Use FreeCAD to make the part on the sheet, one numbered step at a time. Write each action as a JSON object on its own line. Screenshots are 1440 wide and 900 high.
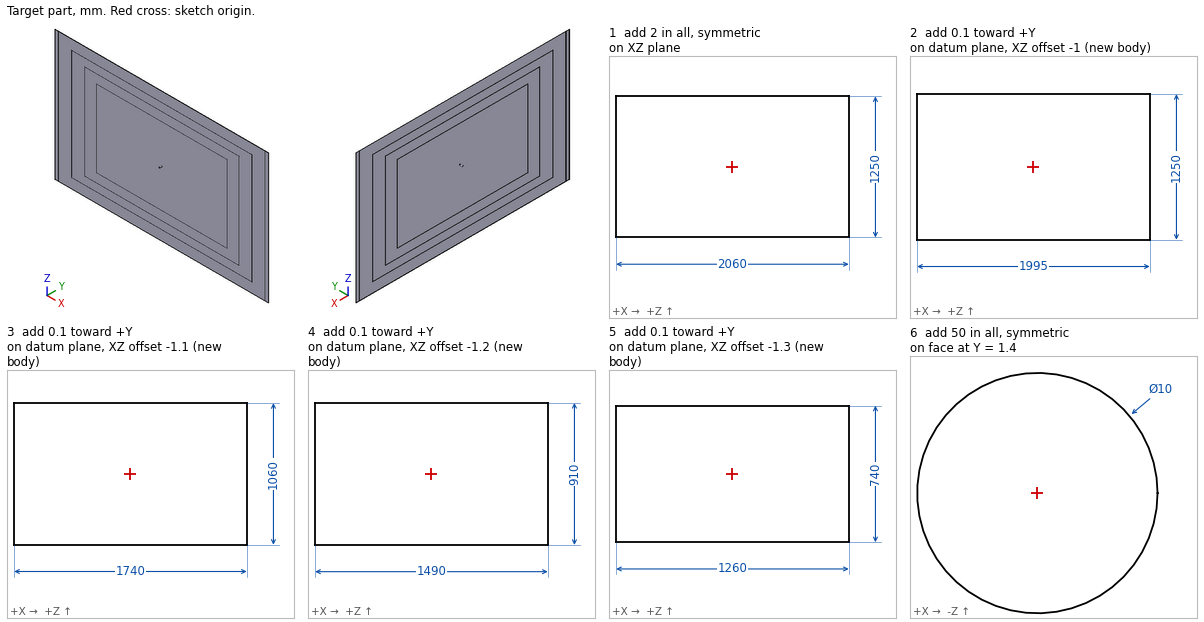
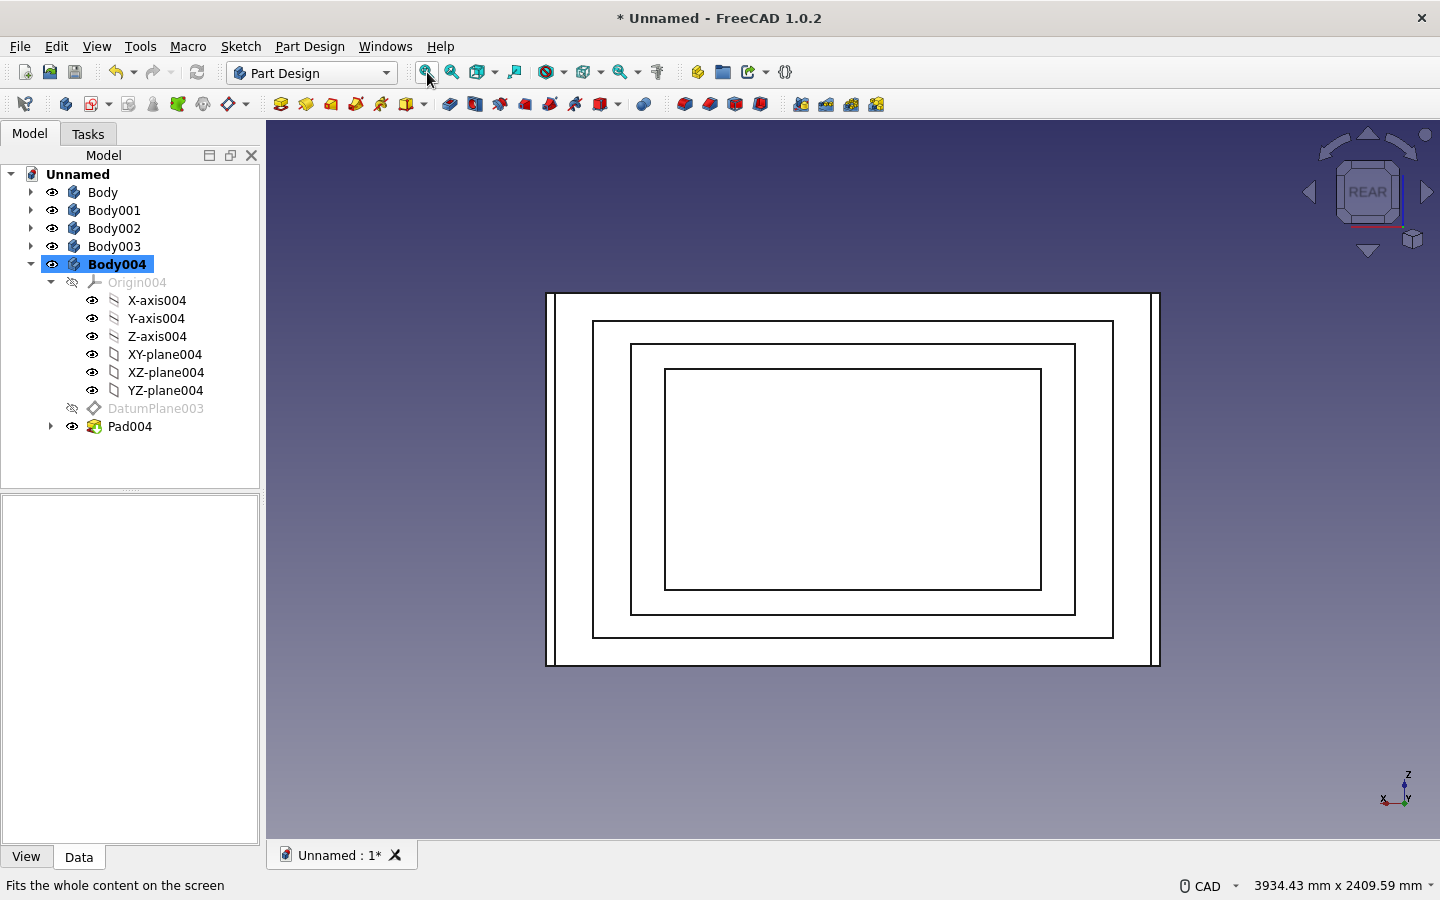
{"action": "left_click", "coordinate": [799, 479]}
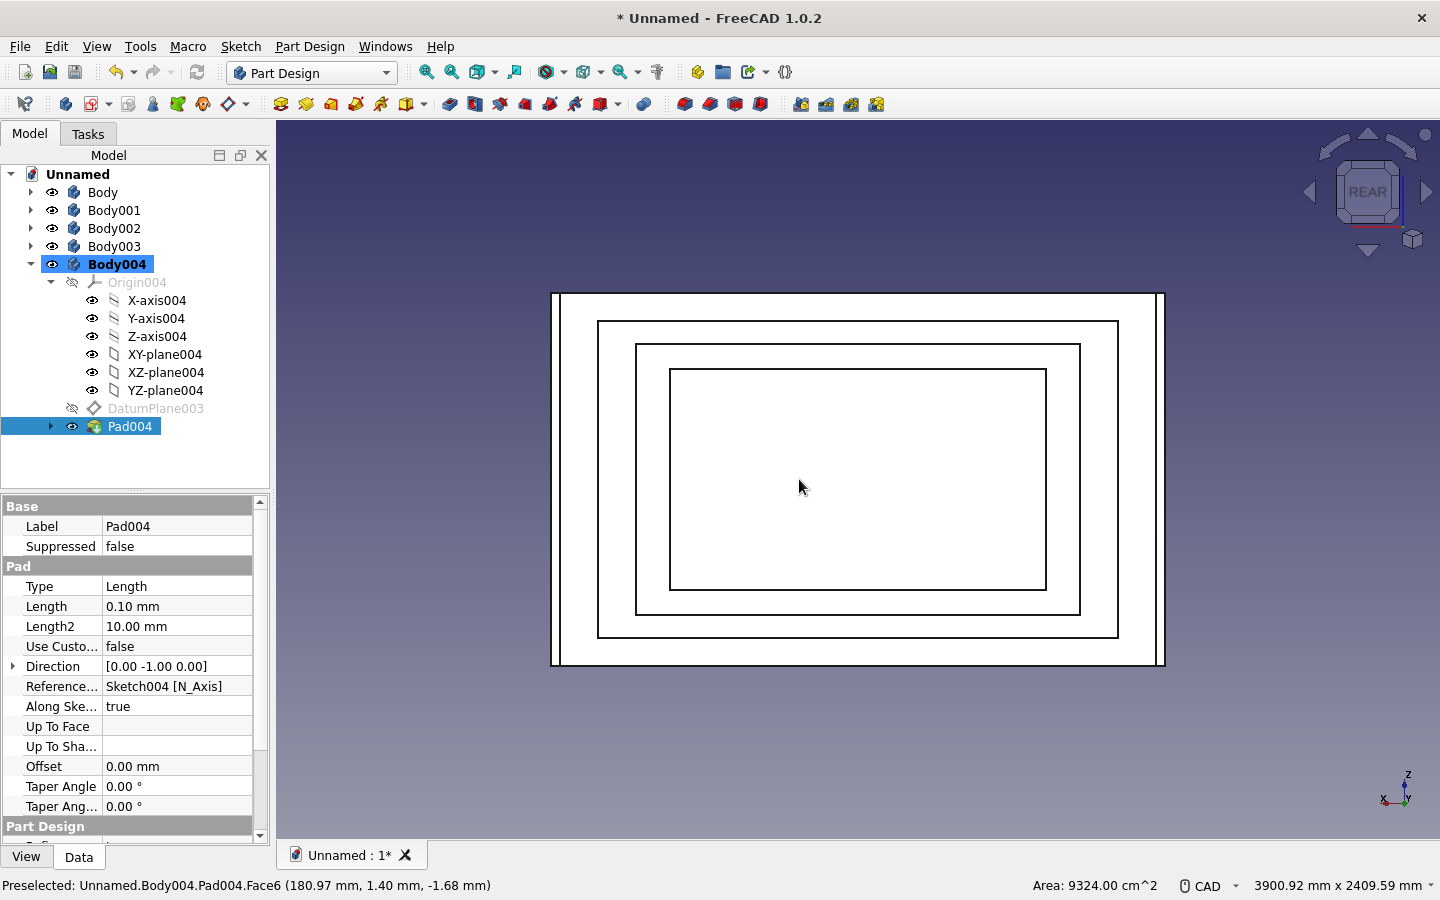
{"action": "left_click", "coordinate": [90, 104]}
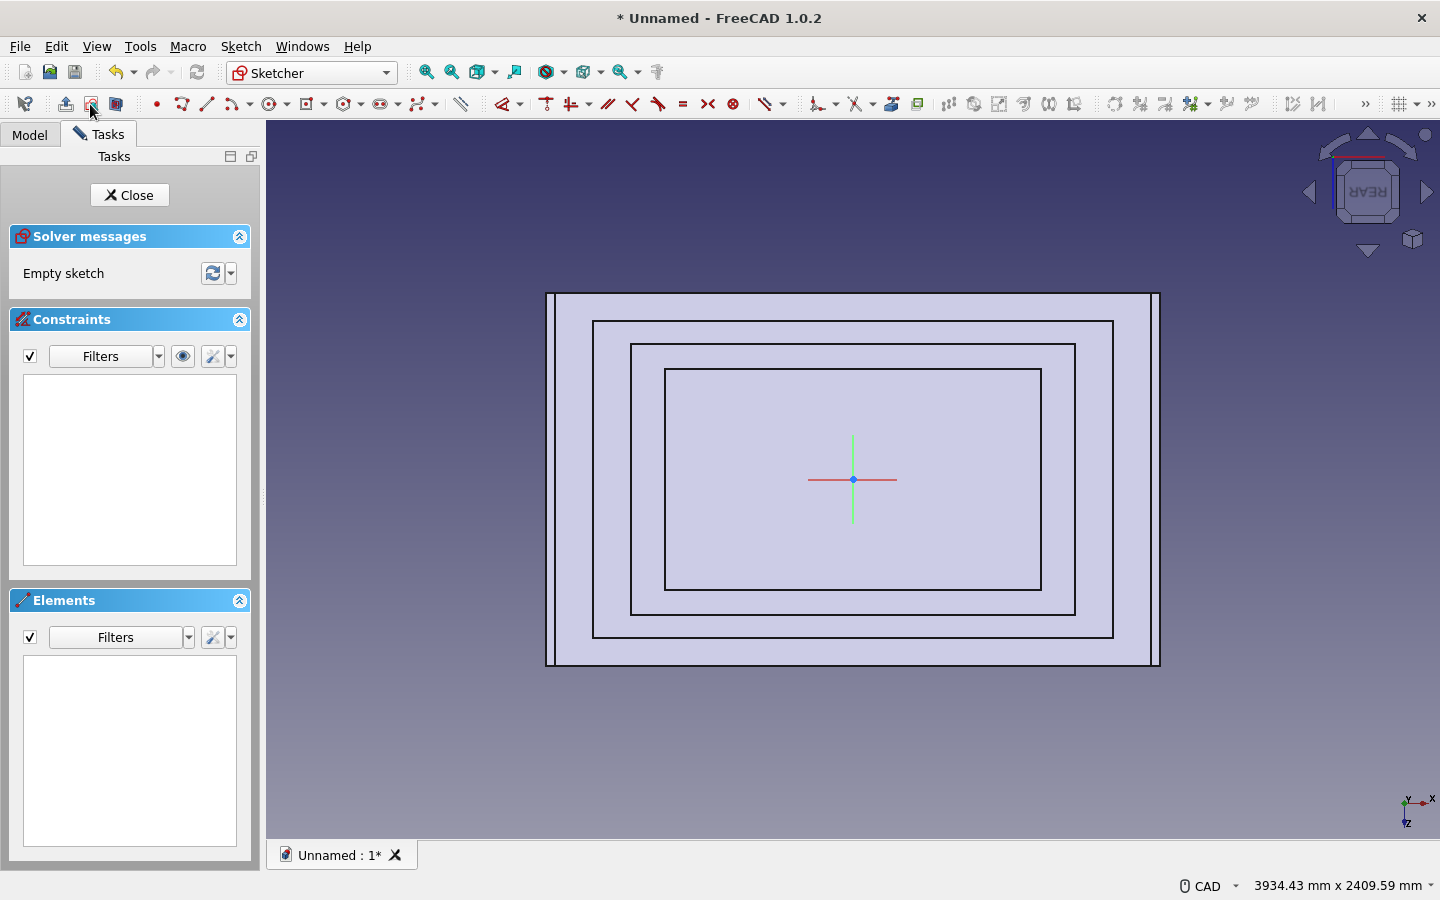
{"action": "scroll", "coordinate": [857, 479], "scroll_direction": "up", "scroll_amount": 15}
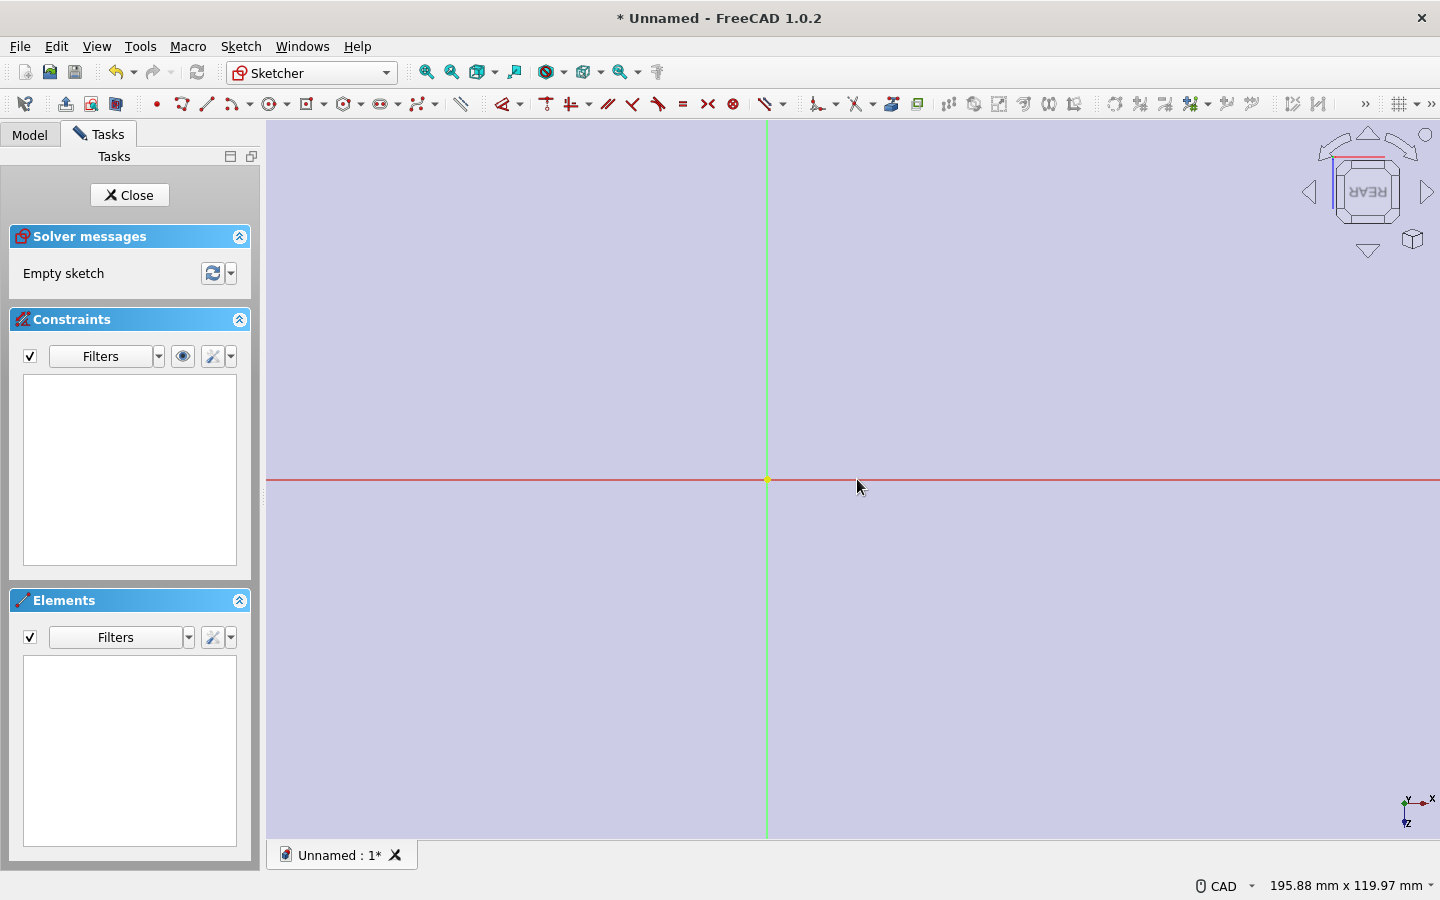
{"action": "scroll", "coordinate": [764, 480], "scroll_direction": "up", "scroll_amount": 10}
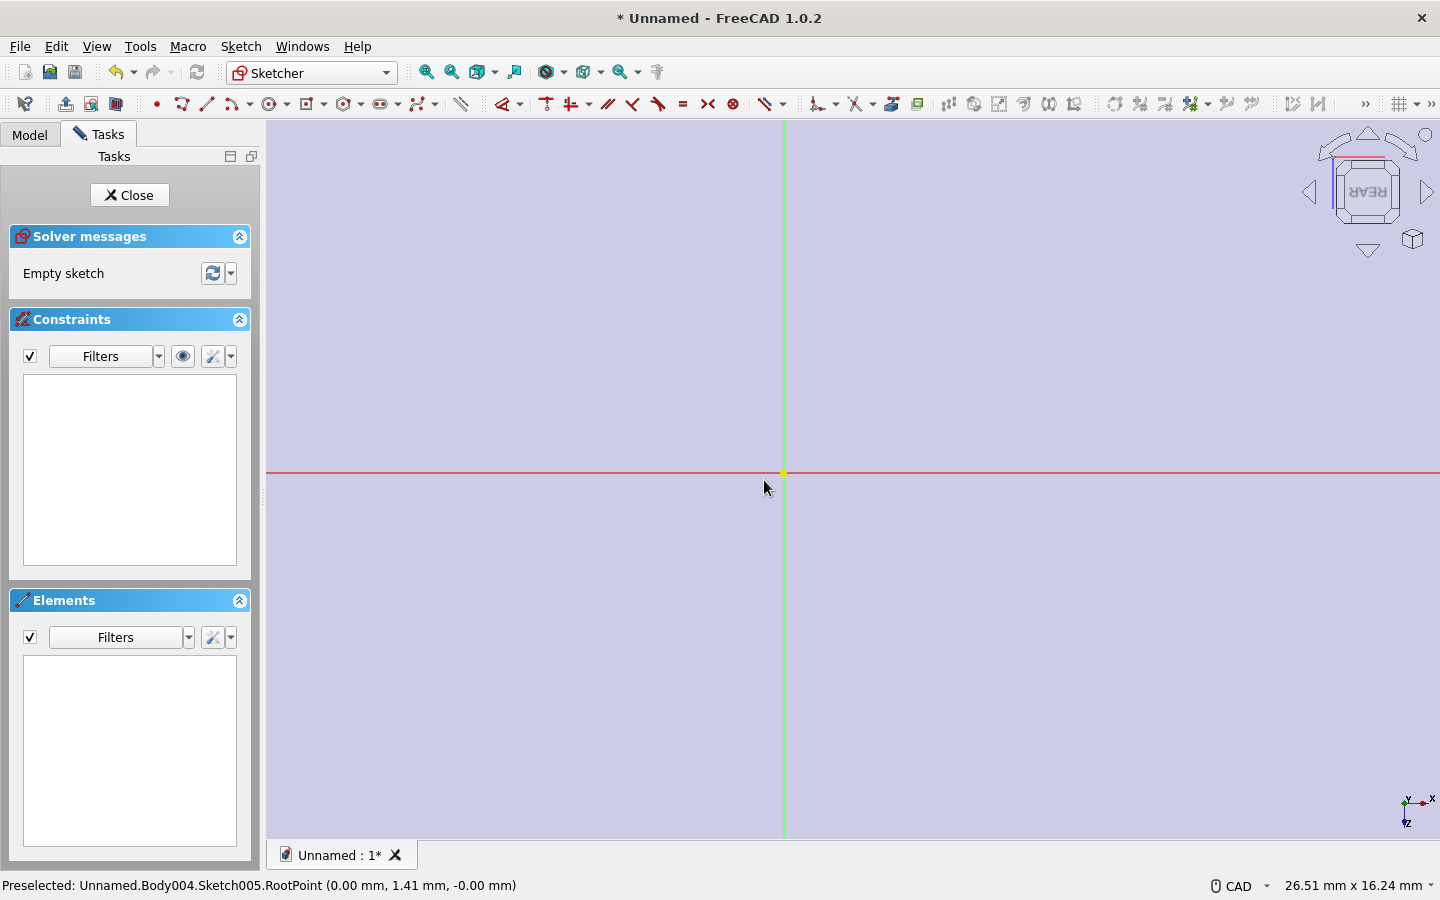
{"action": "left_click", "coordinate": [268, 104]}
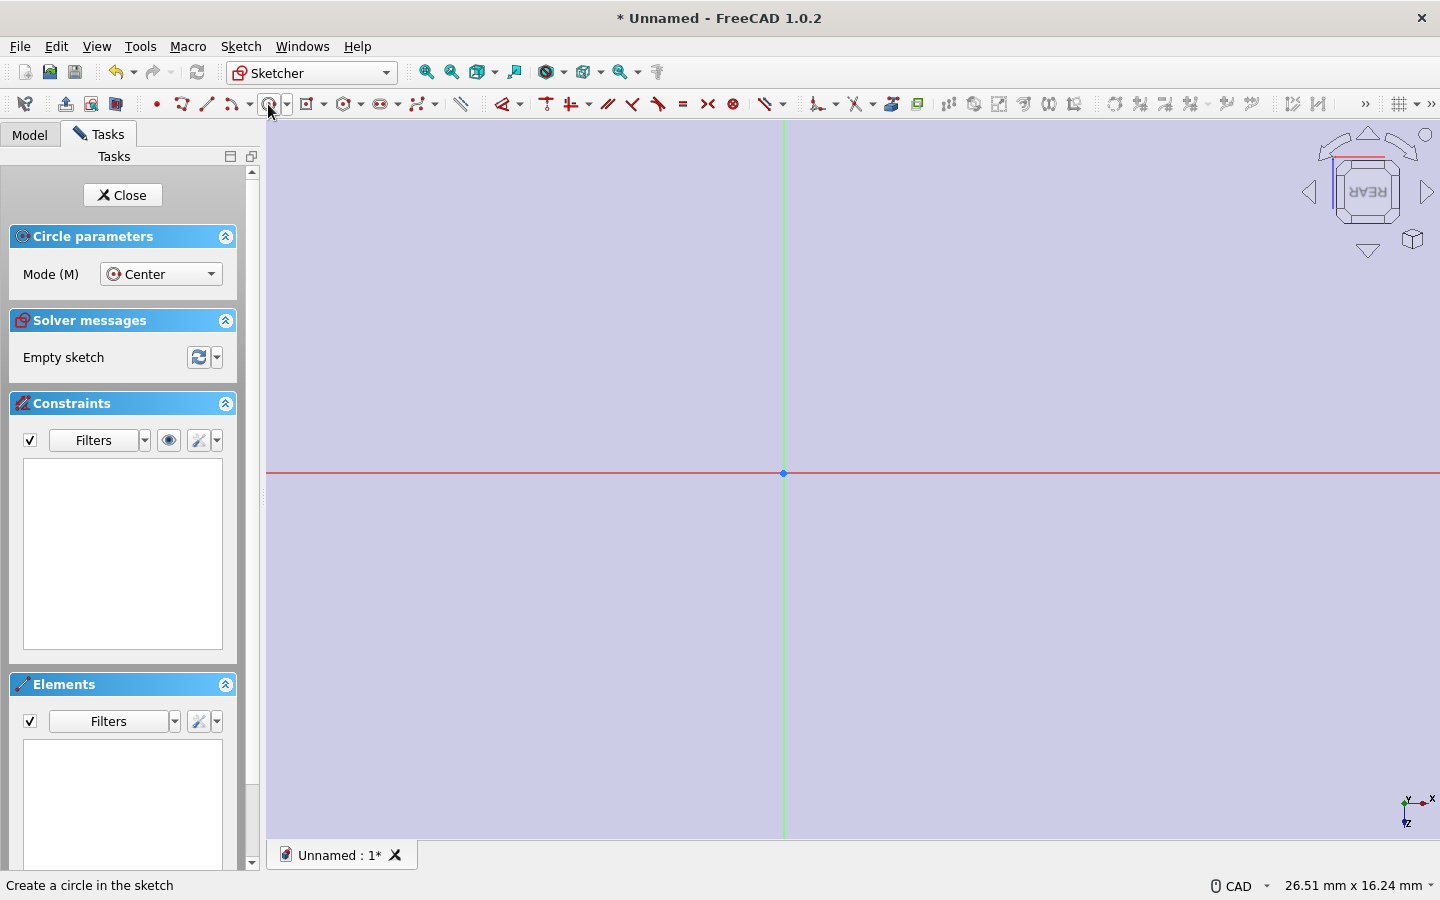
{"action": "left_click", "coordinate": [784, 473]}
{"action": "mouse_move", "coordinate": [940, 317]}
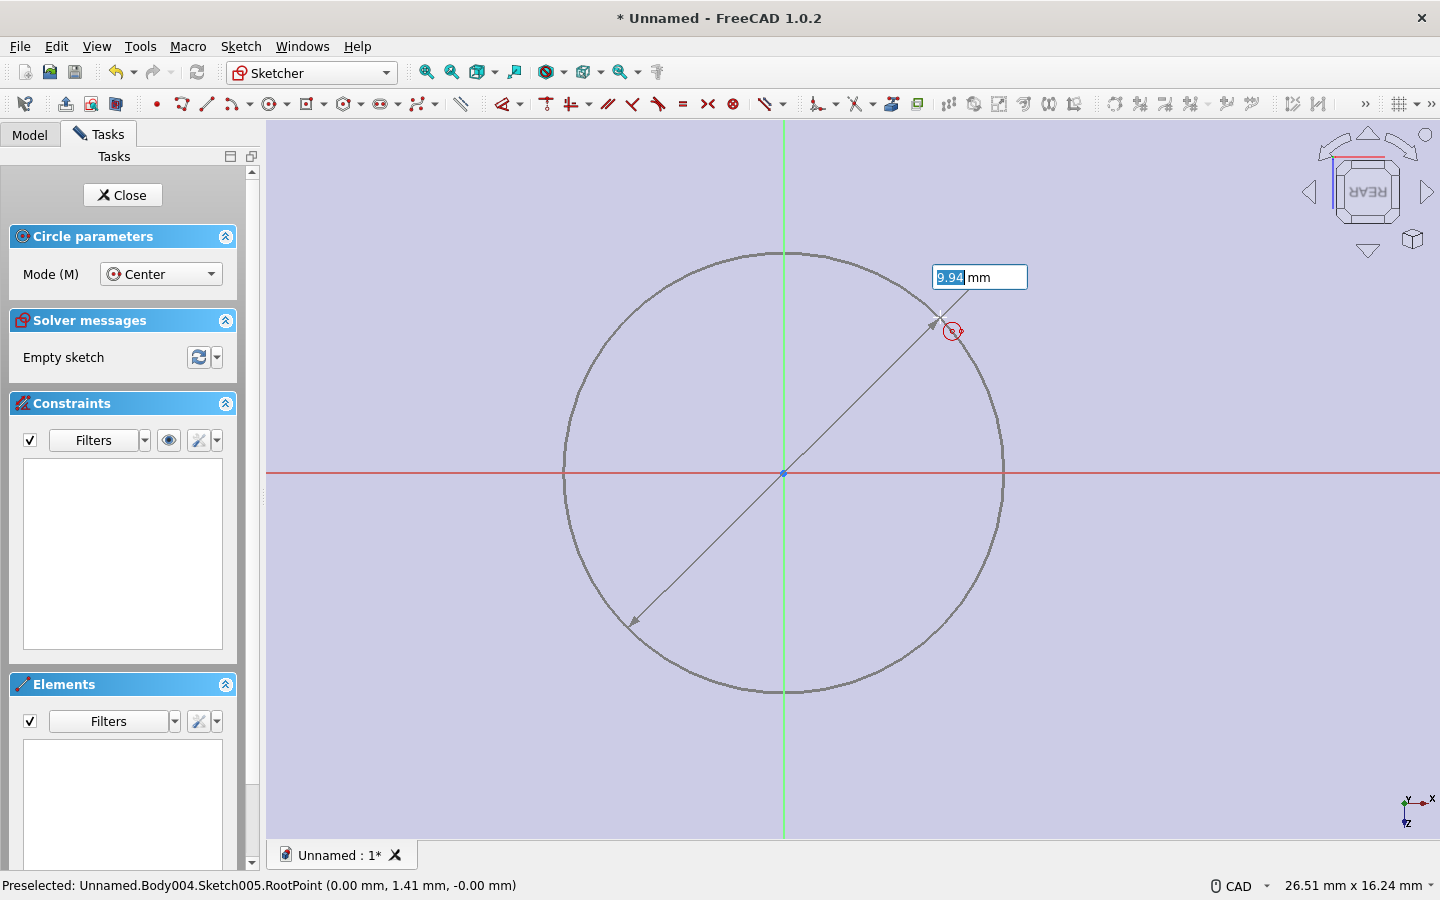
{"action": "type", "text": "10"}
{"action": "key", "text": "Return"}
{"action": "key", "text": "Escape"}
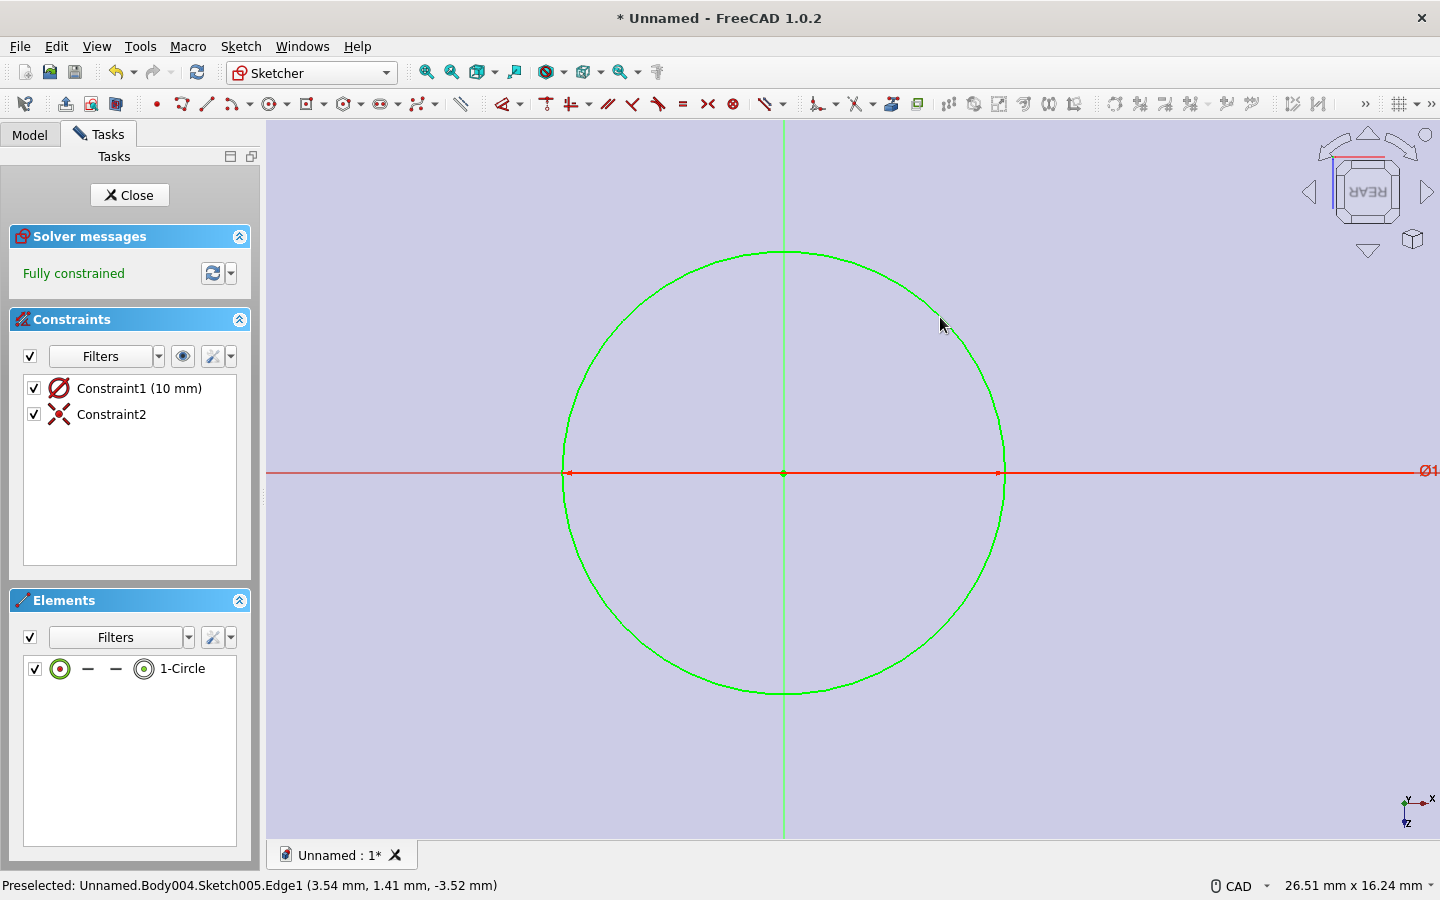
{"action": "left_click", "coordinate": [130, 195]}